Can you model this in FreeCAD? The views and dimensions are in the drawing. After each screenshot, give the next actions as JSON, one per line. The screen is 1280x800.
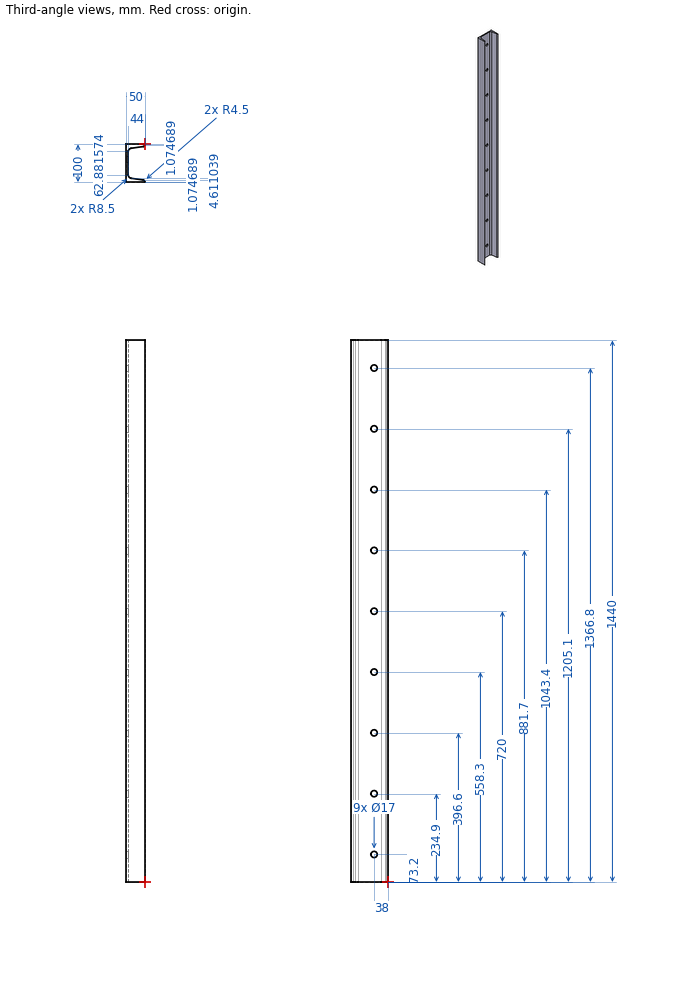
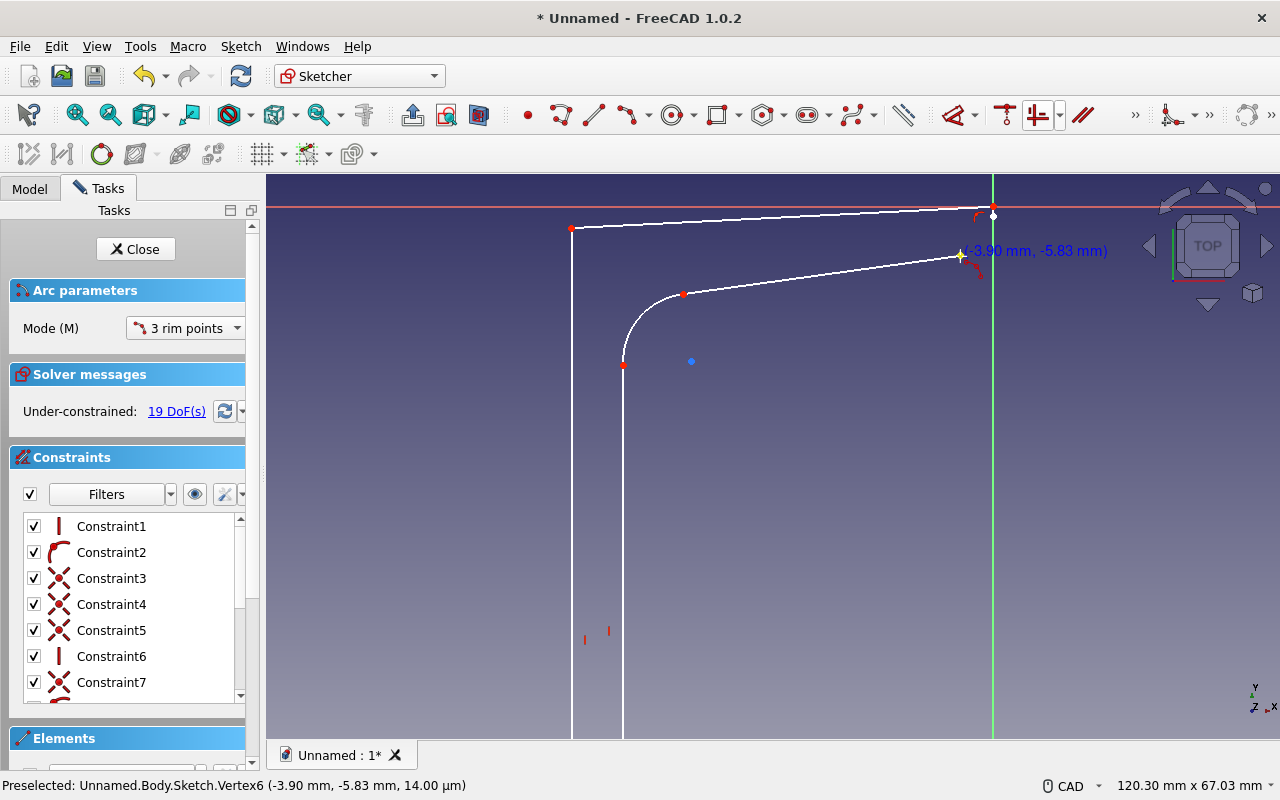
{"action": "scroll", "coordinate": [993, 216], "scroll_direction": "up", "scroll_amount": 7}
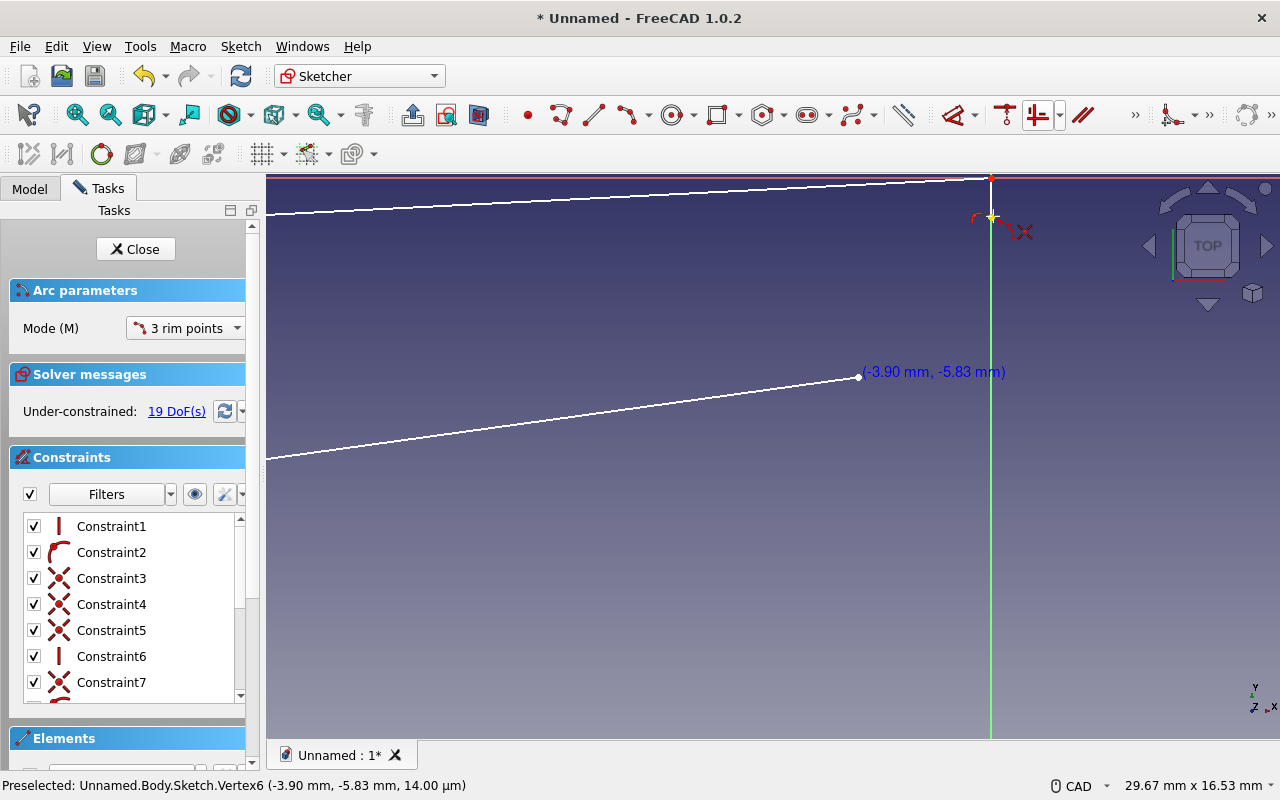
{"action": "left_click", "coordinate": [991, 217]}
{"action": "left_click", "coordinate": [954, 316]}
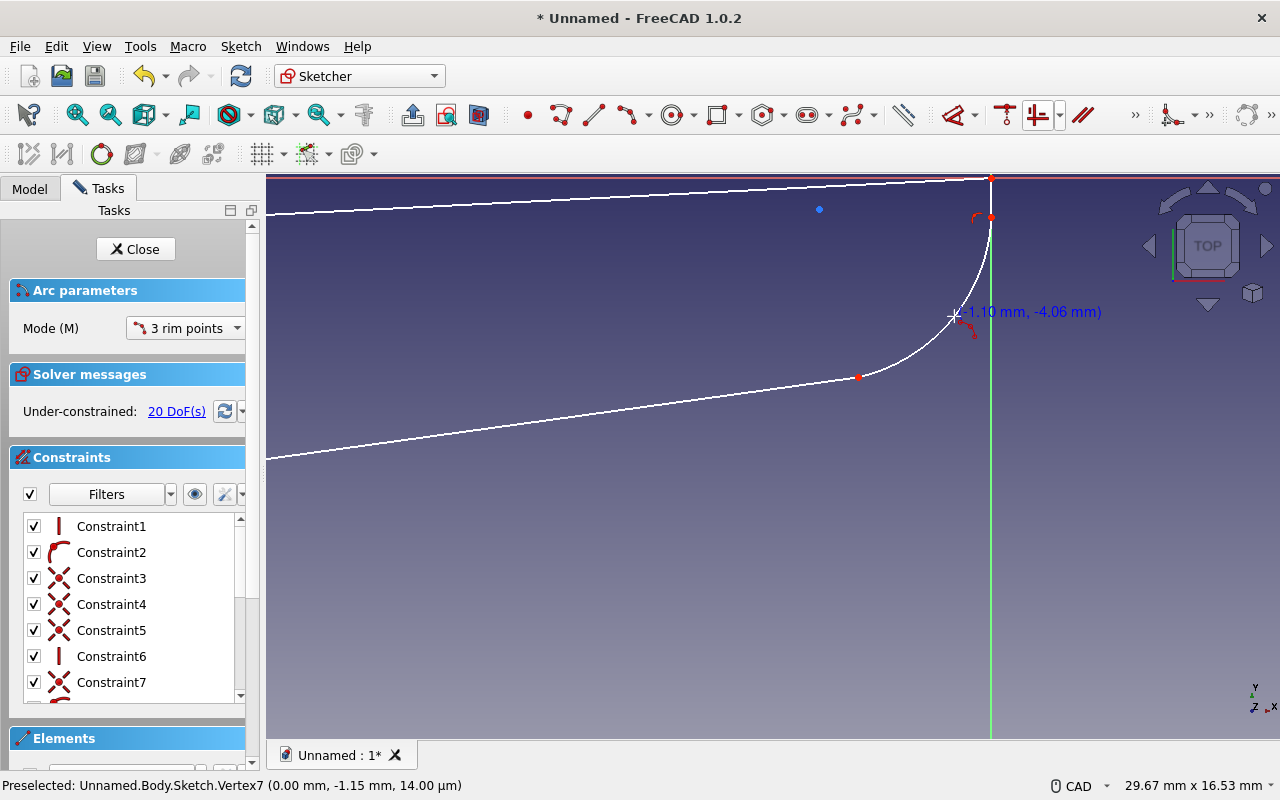
{"action": "scroll", "coordinate": [775, 278], "scroll_direction": "down", "scroll_amount": 11}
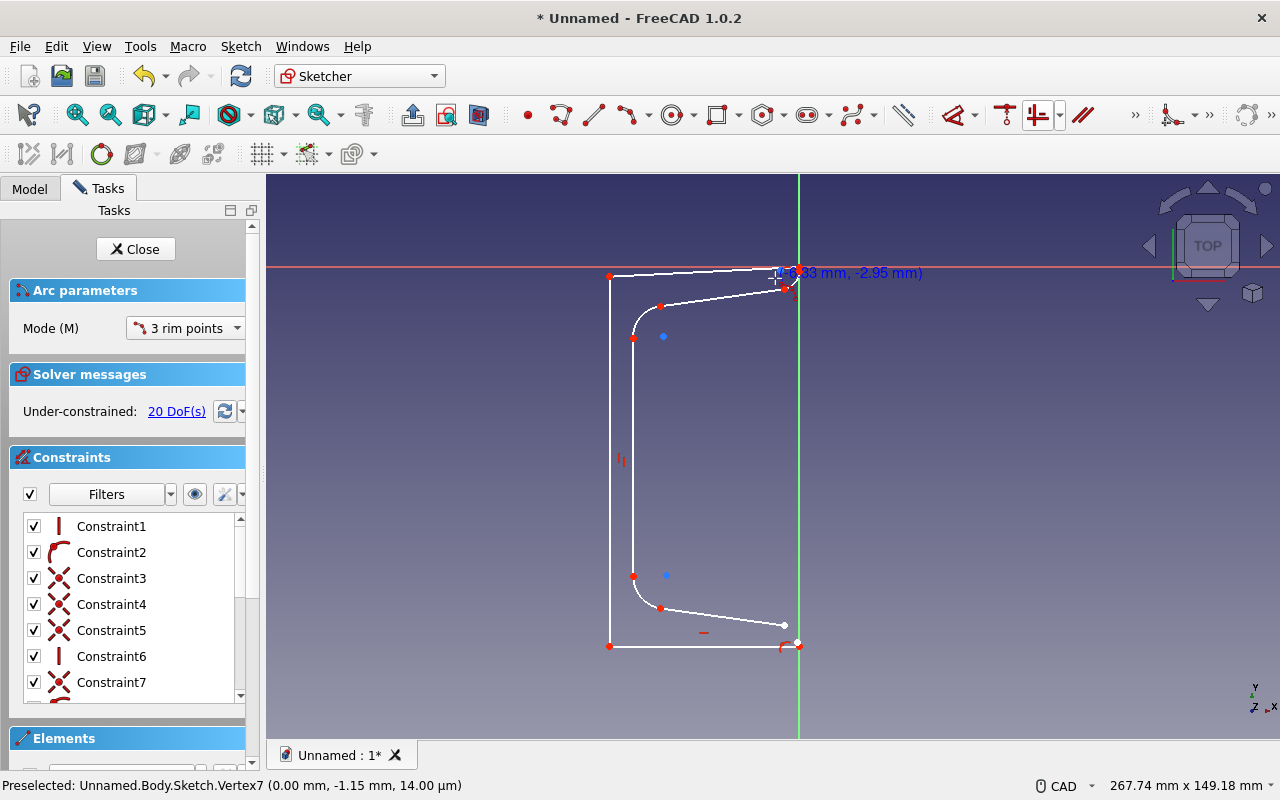
{"action": "scroll", "coordinate": [799, 642], "scroll_direction": "up", "scroll_amount": 11}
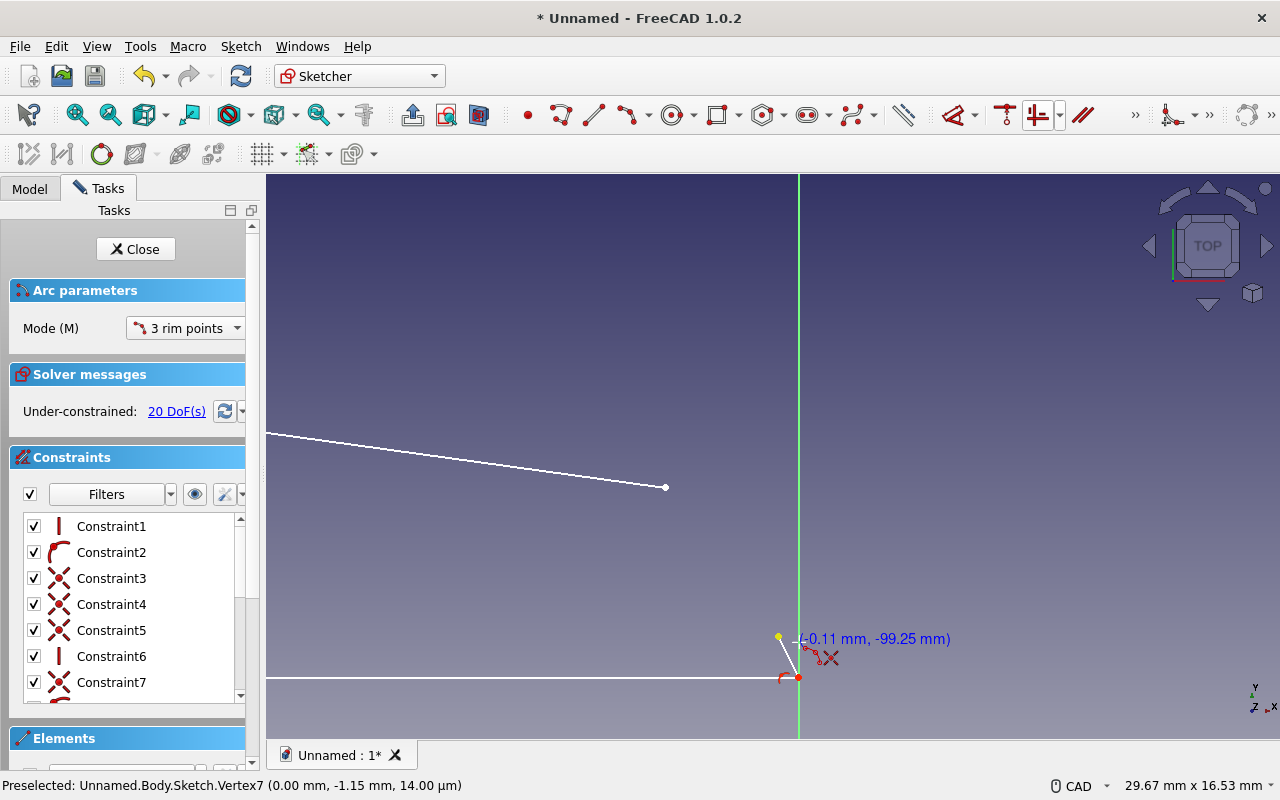
{"action": "left_click", "coordinate": [778, 636]}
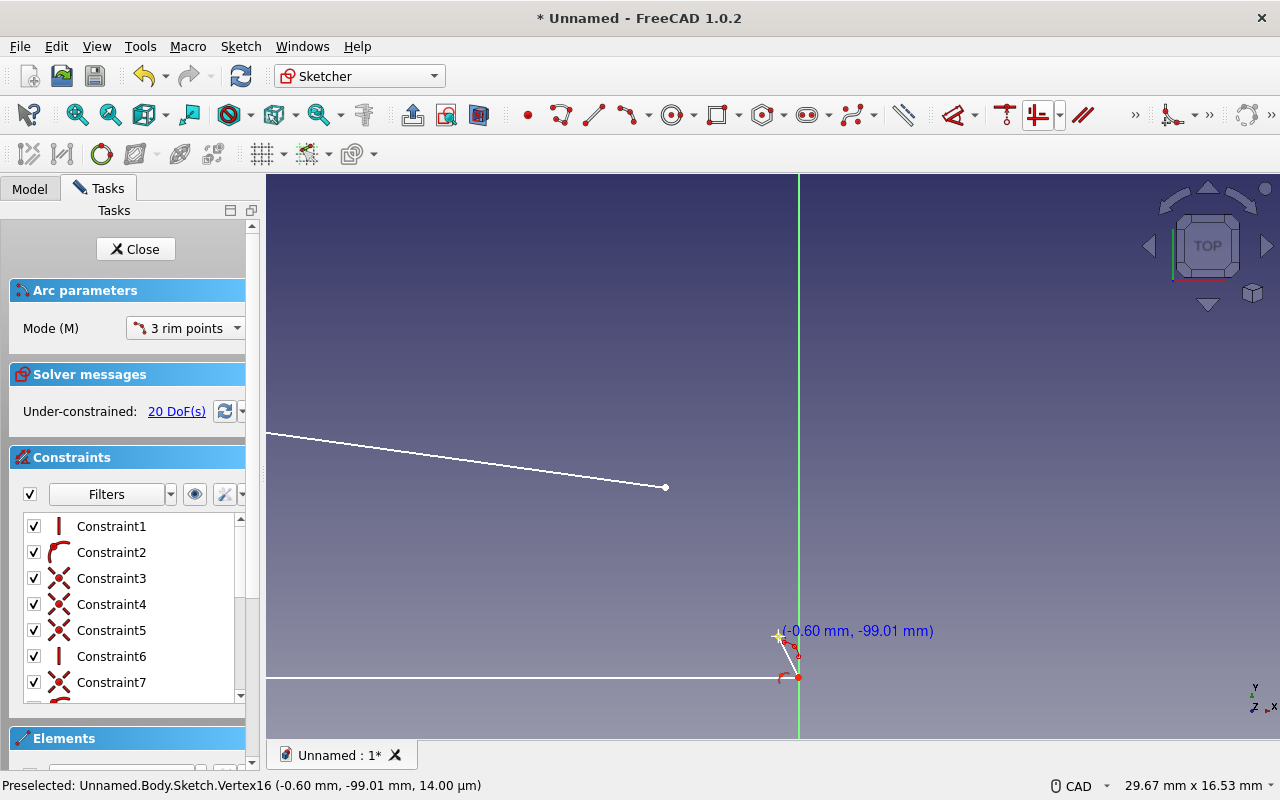
{"action": "scroll", "coordinate": [799, 643], "scroll_direction": "down", "scroll_amount": 11}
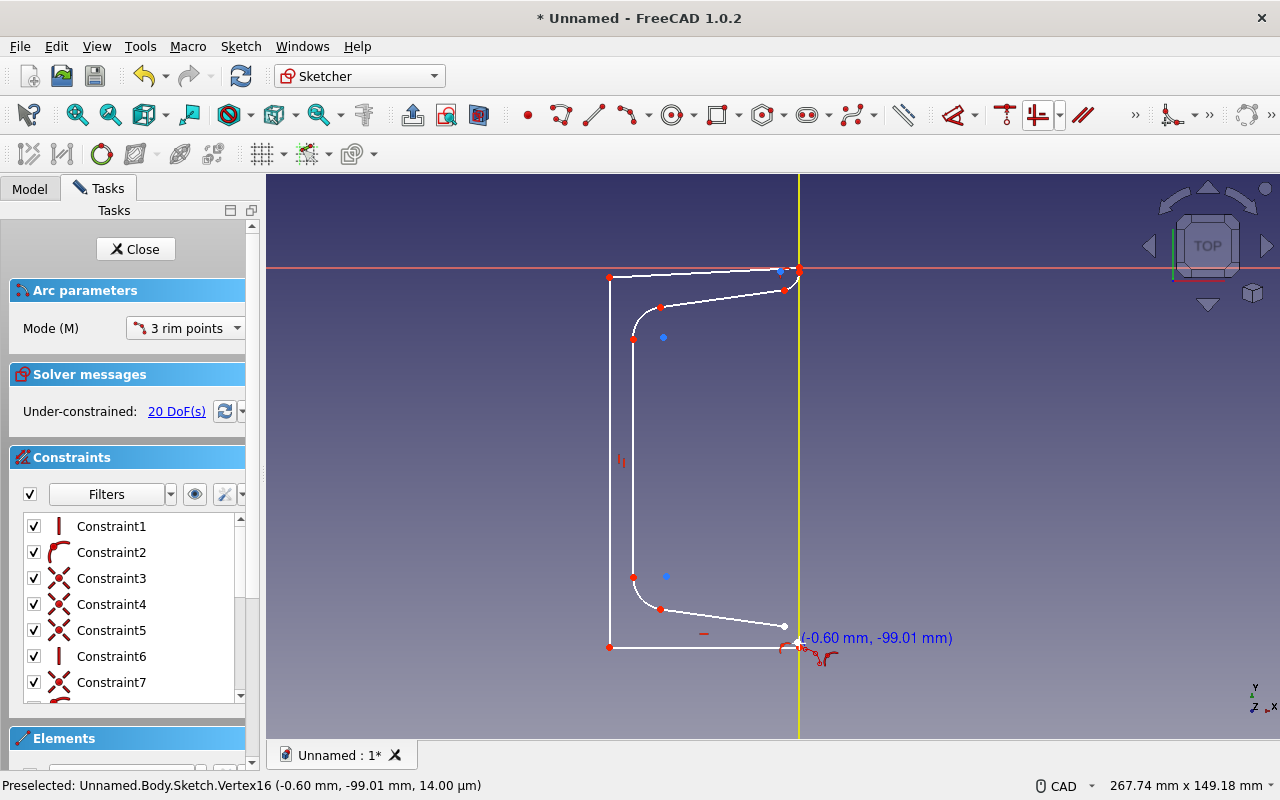
{"action": "left_click", "coordinate": [785, 627]}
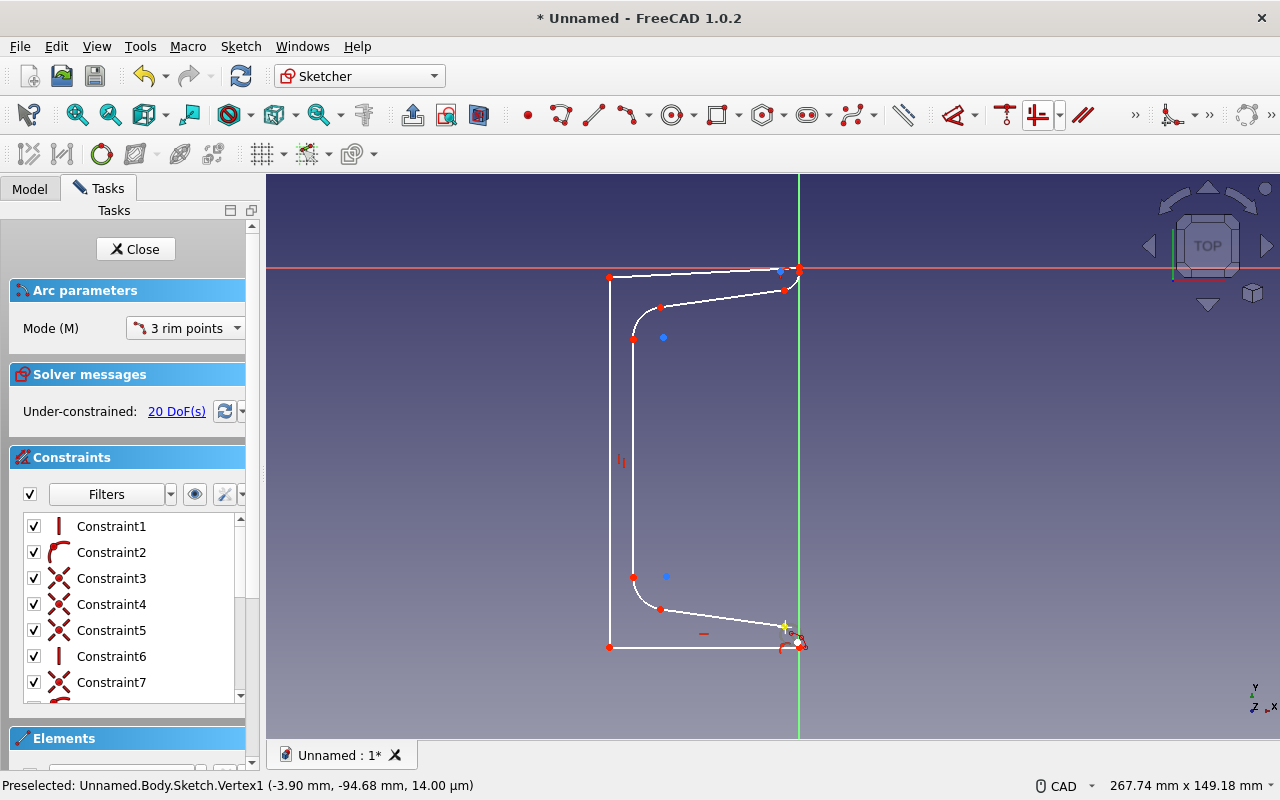
{"action": "scroll", "coordinate": [795, 631], "scroll_direction": "up", "scroll_amount": 7}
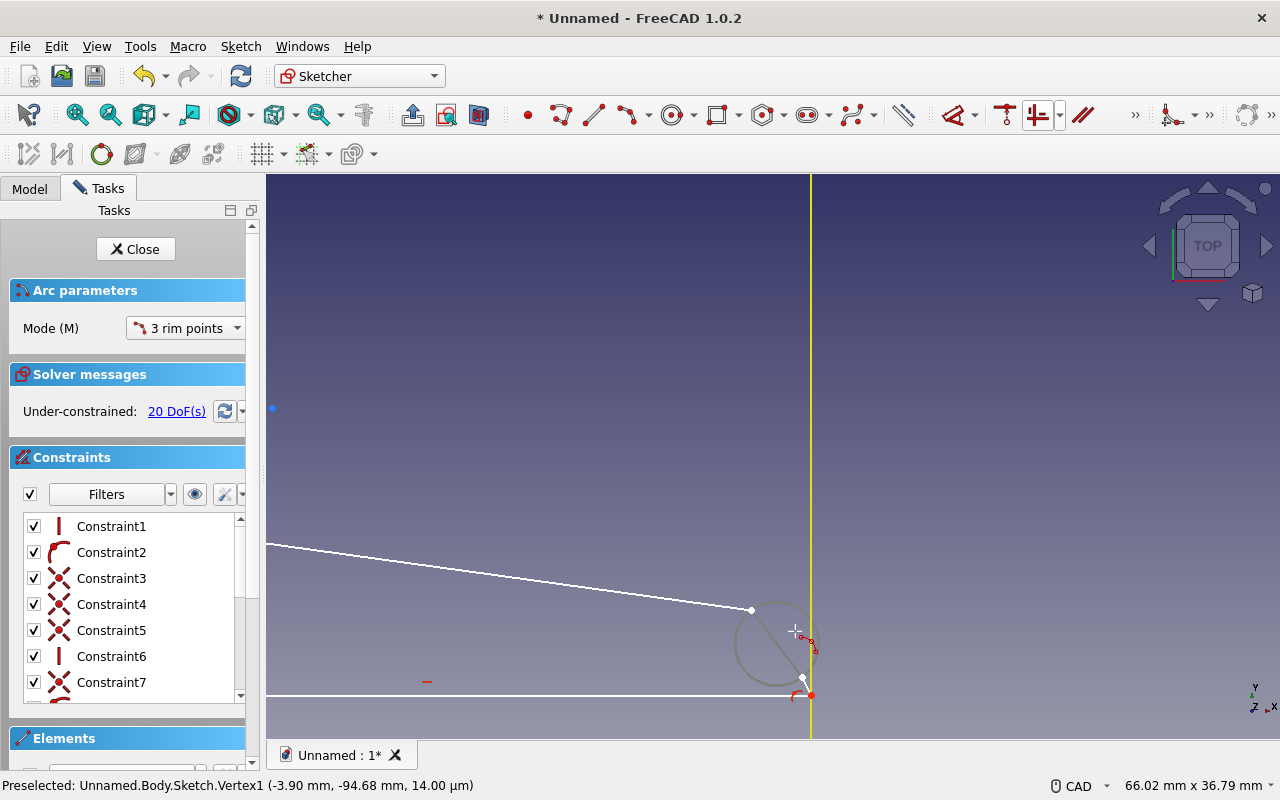
{"action": "left_click", "coordinate": [794, 630]}
{"action": "key", "text": "Escape"}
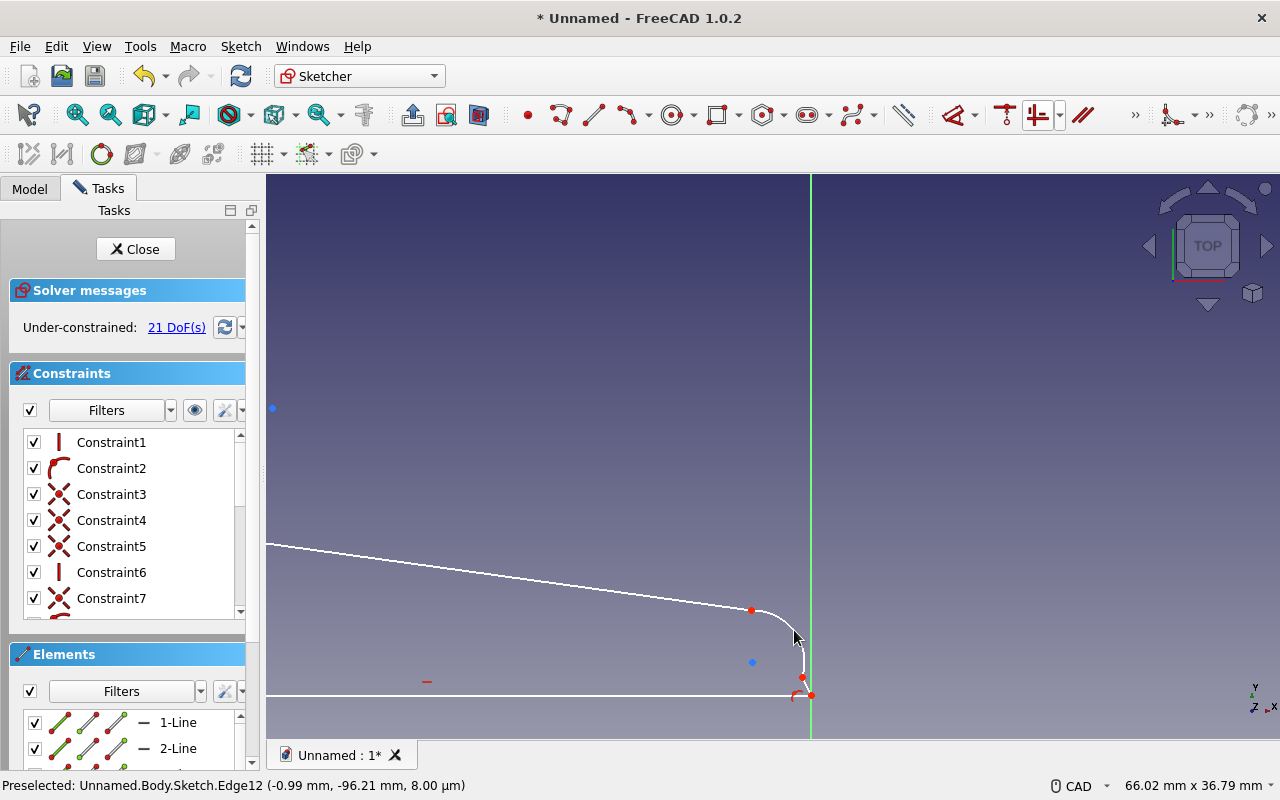
{"action": "scroll", "coordinate": [795, 631], "scroll_direction": "down", "scroll_amount": 7}